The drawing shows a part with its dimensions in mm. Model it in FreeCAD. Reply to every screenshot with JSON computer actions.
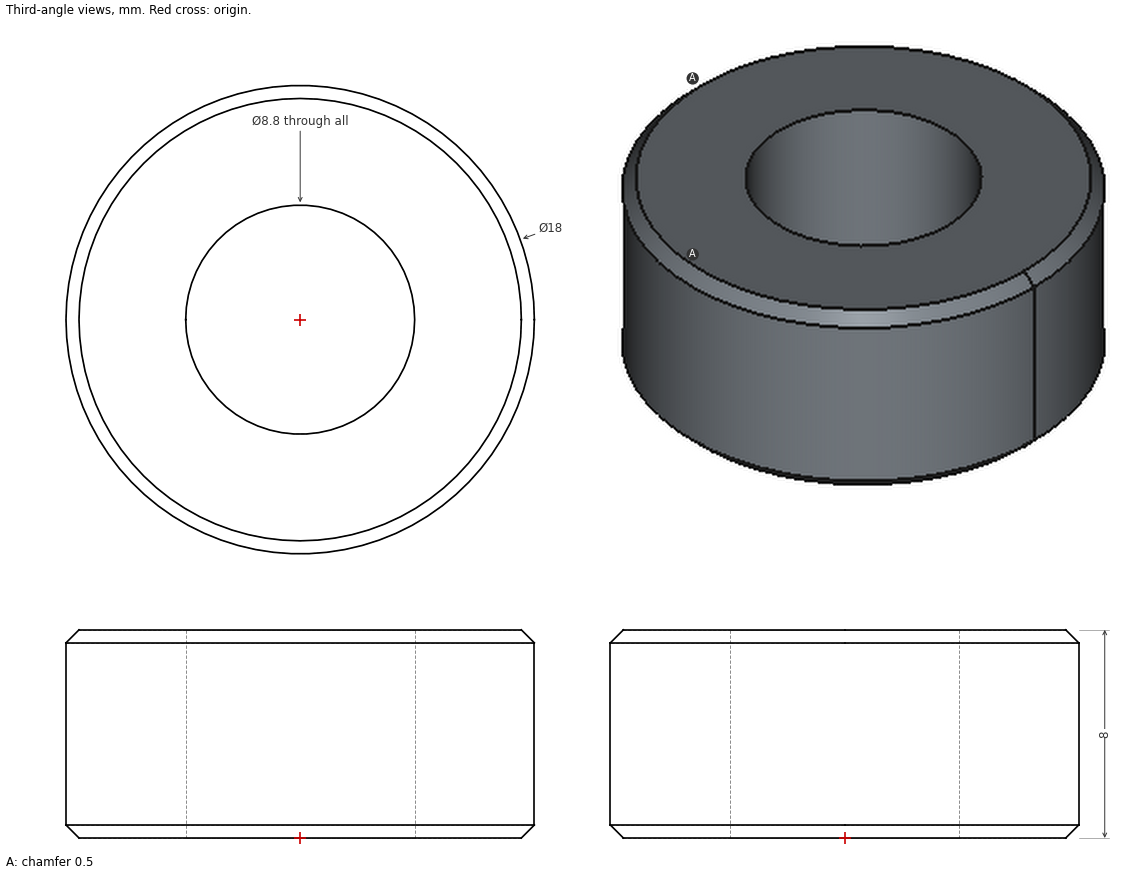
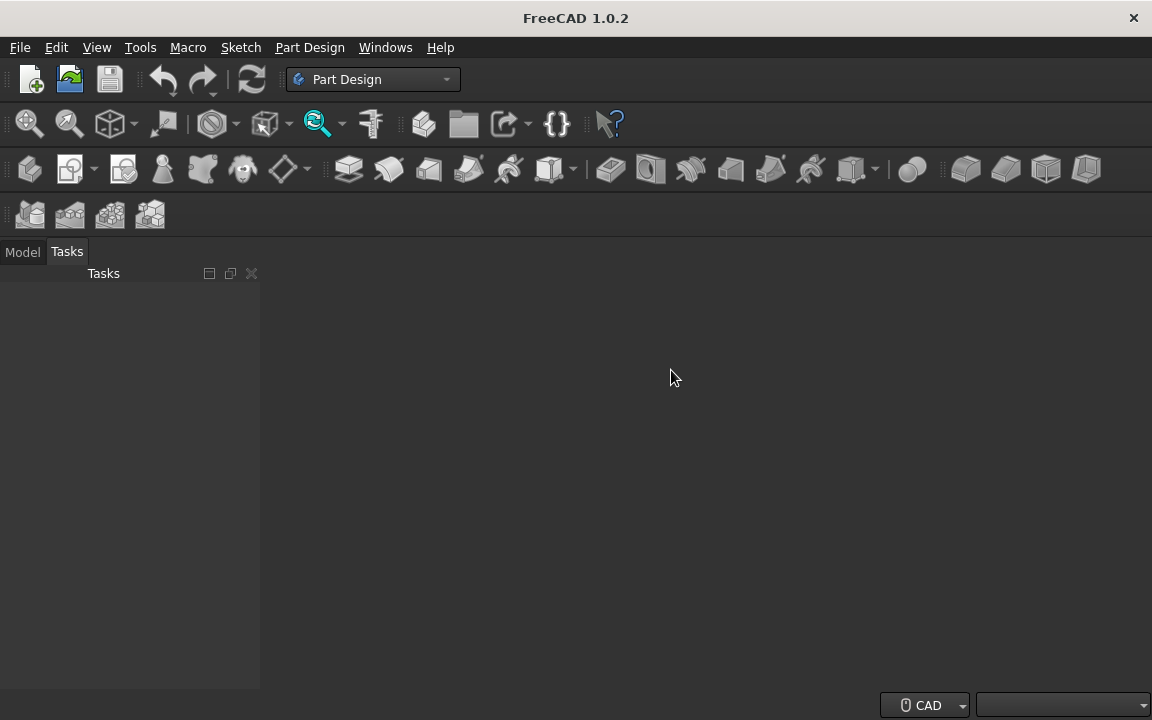
{"action": "left_click", "coordinate": [30, 80]}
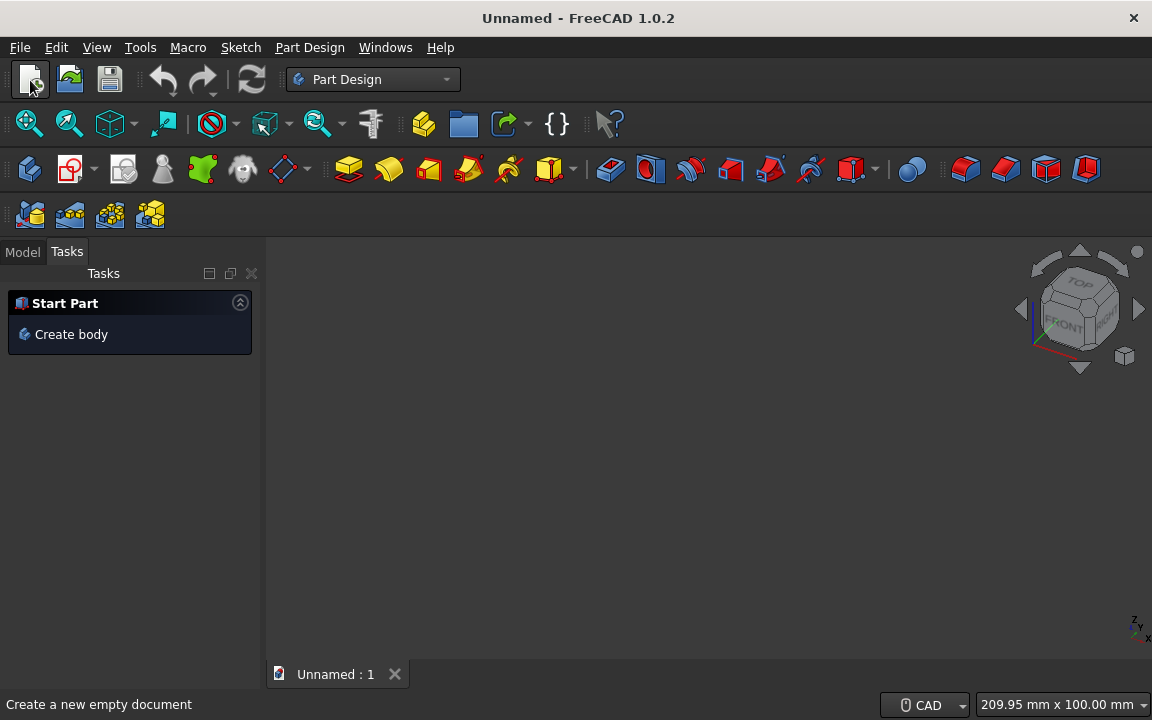
{"action": "left_click", "coordinate": [70, 170]}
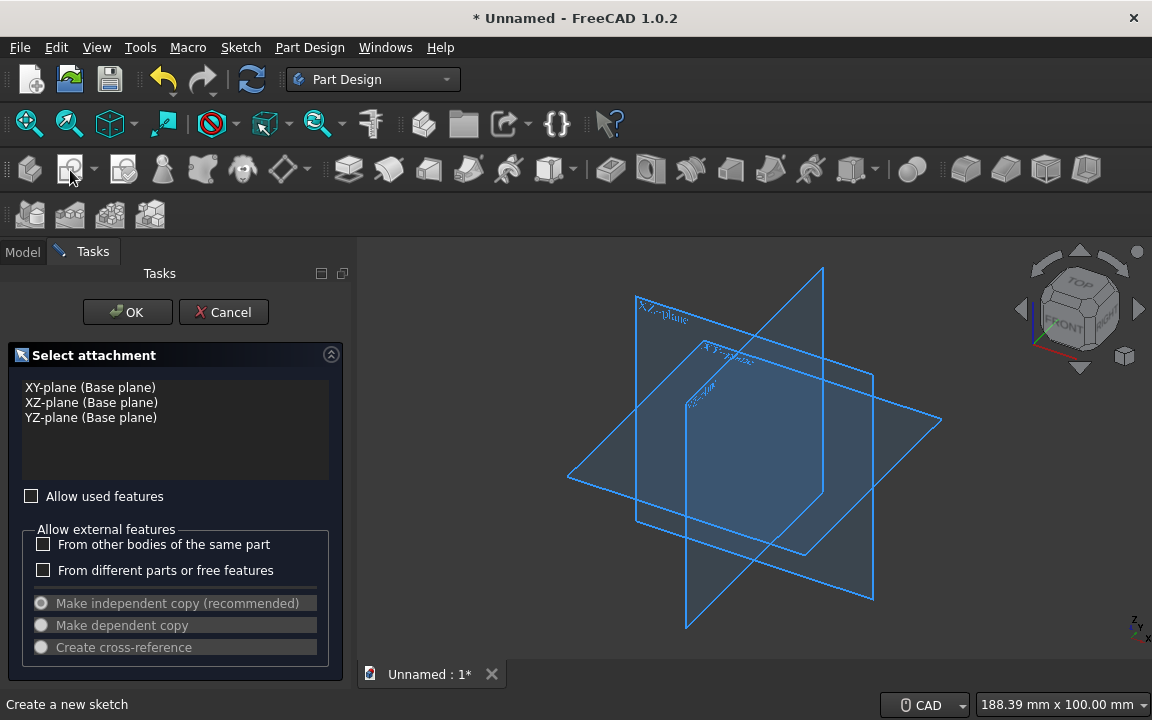
{"action": "left_click", "coordinate": [82, 388]}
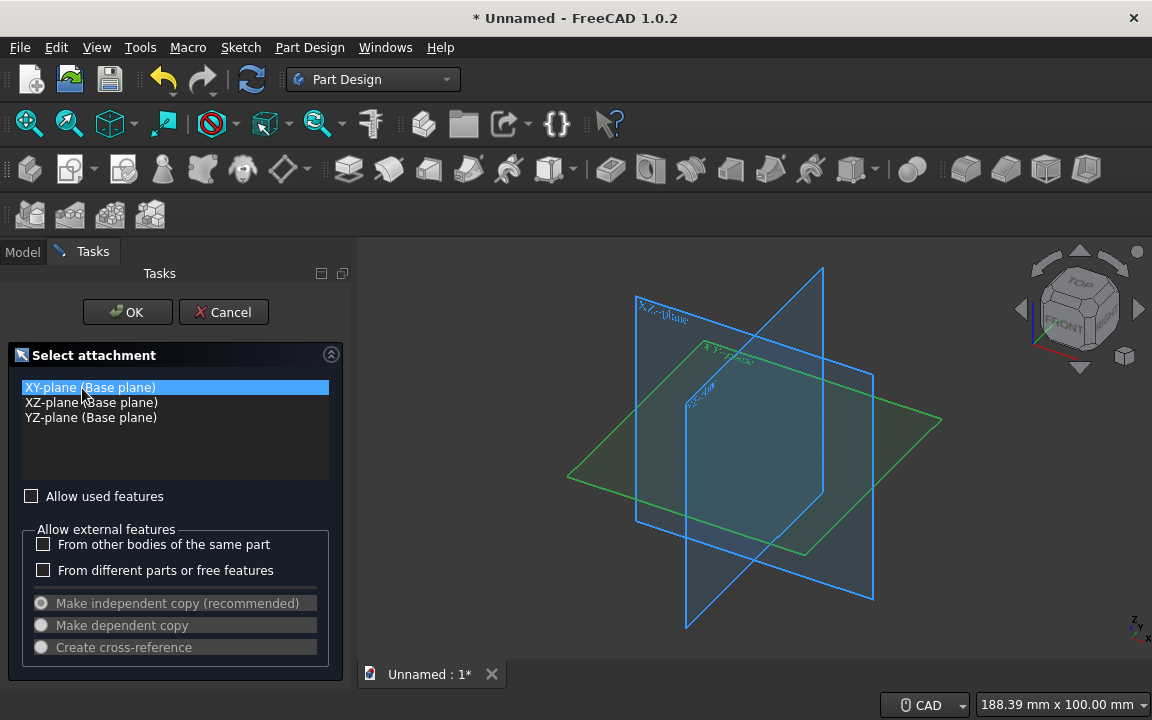
{"action": "left_click", "coordinate": [128, 312]}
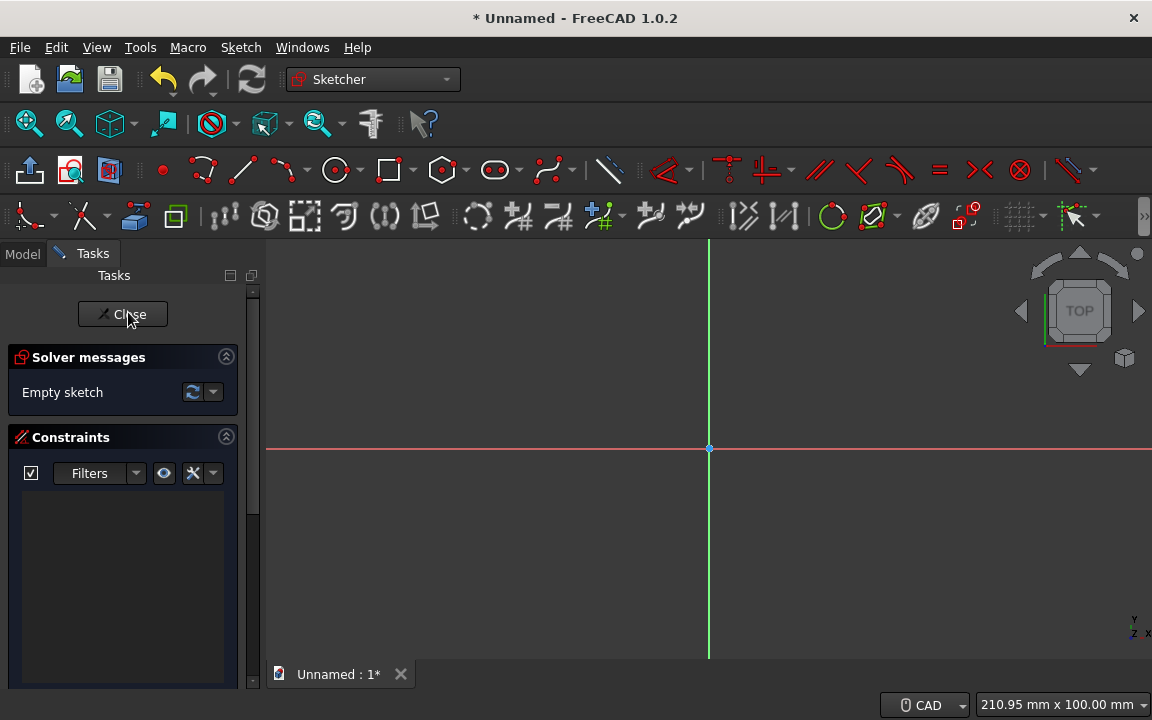
{"action": "scroll", "coordinate": [739, 449], "scroll_direction": "up", "scroll_amount": 6}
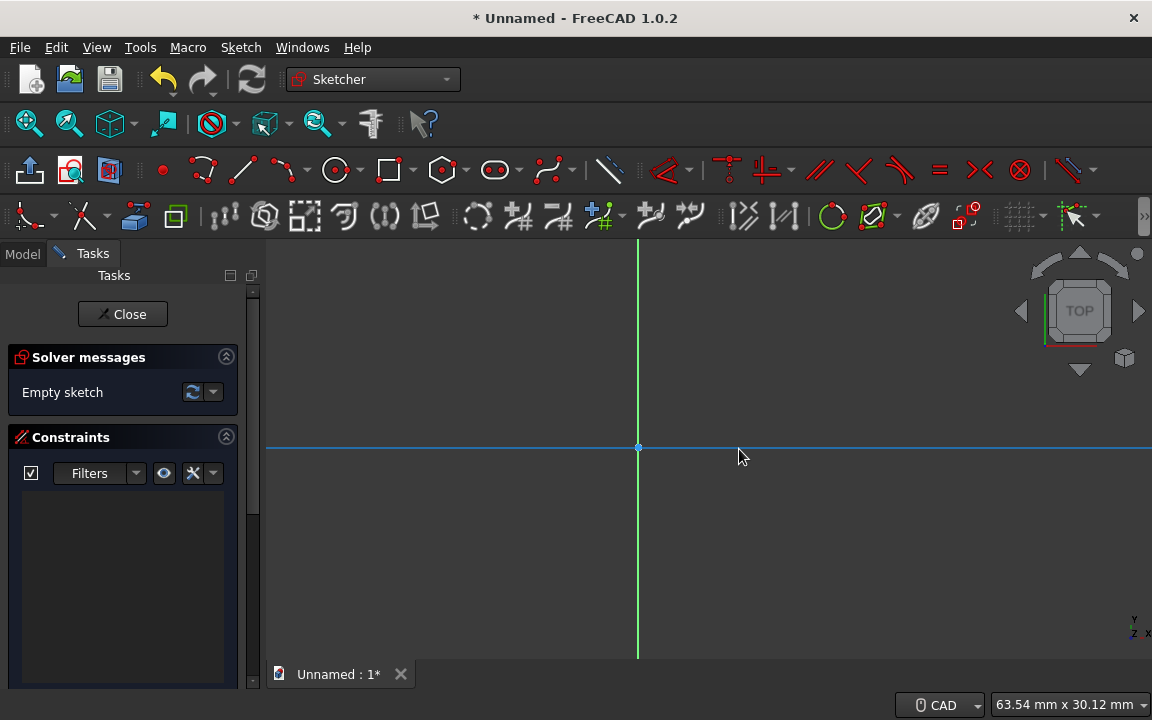
{"action": "left_click", "coordinate": [336, 170]}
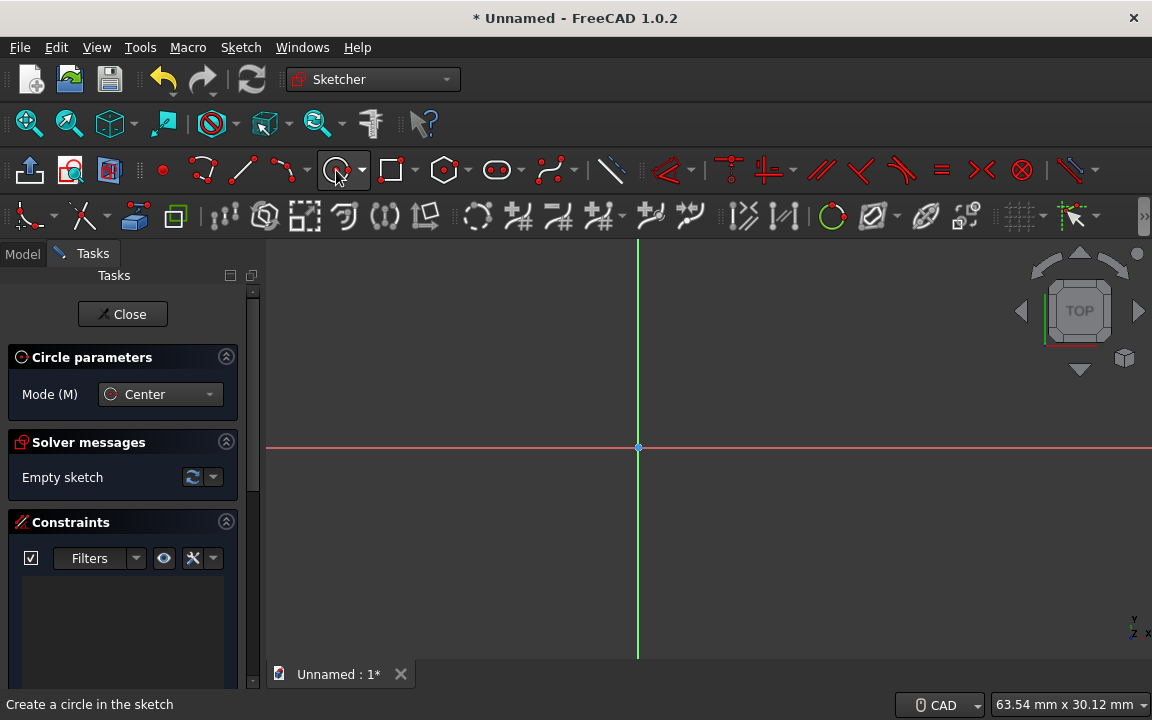
{"action": "left_click", "coordinate": [638, 448]}
{"action": "left_click", "coordinate": [727, 359]}
{"action": "key", "text": "Escape"}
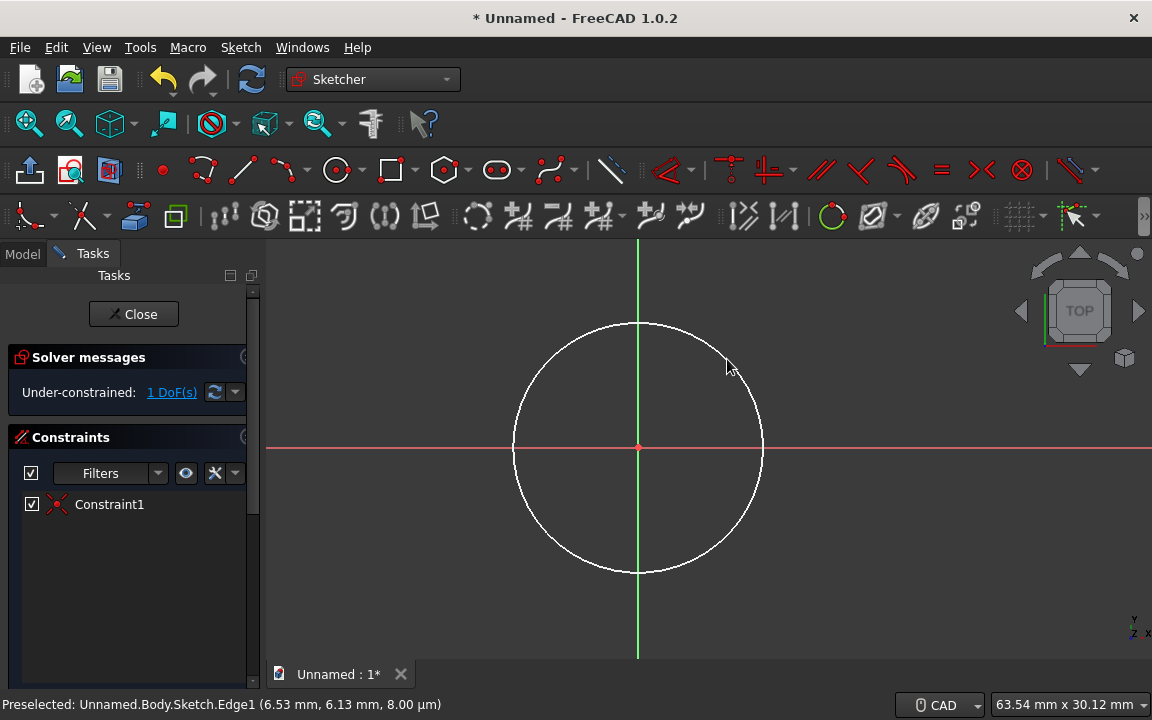
{"action": "key", "text": "d"}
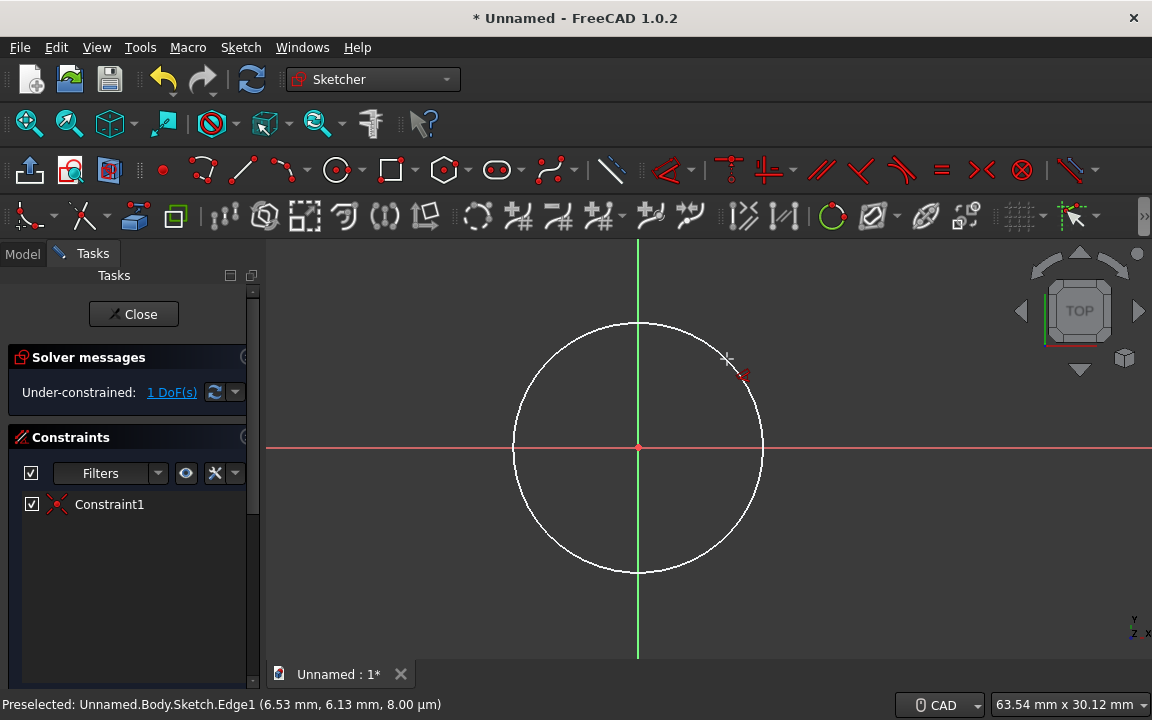
{"action": "left_click", "coordinate": [726, 359]}
{"action": "left_click", "coordinate": [748, 336]}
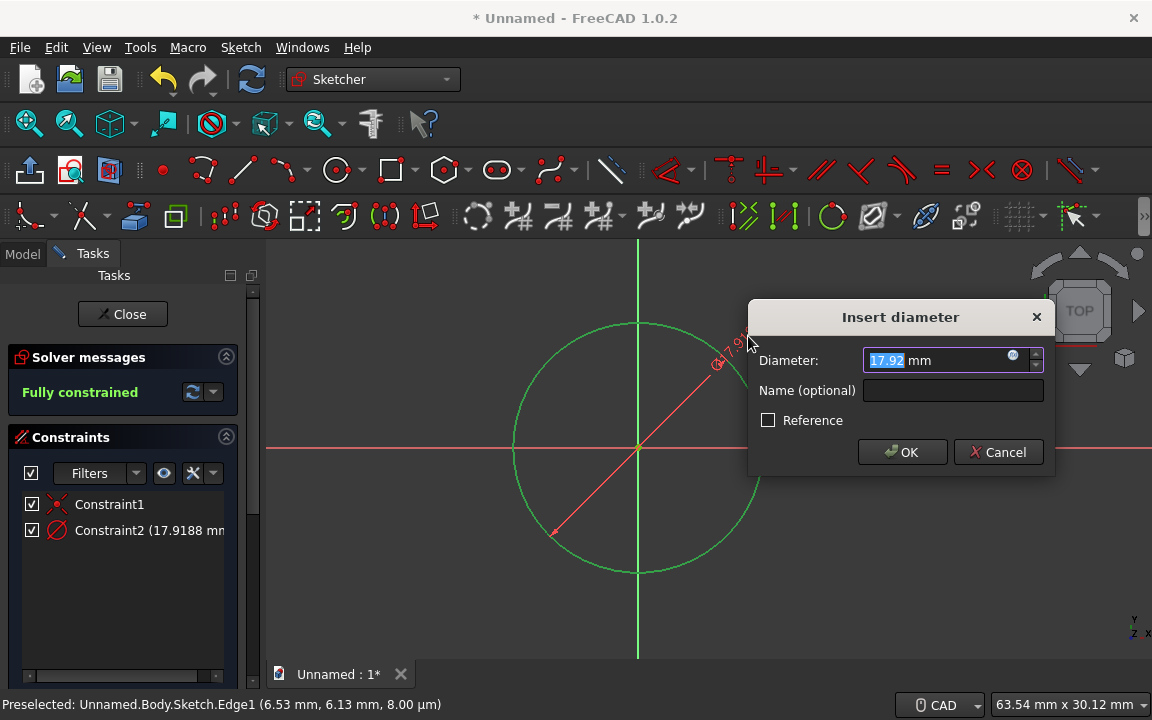
{"action": "type", "text": "18"}
{"action": "key", "text": "Return"}
{"action": "key", "text": "Escape"}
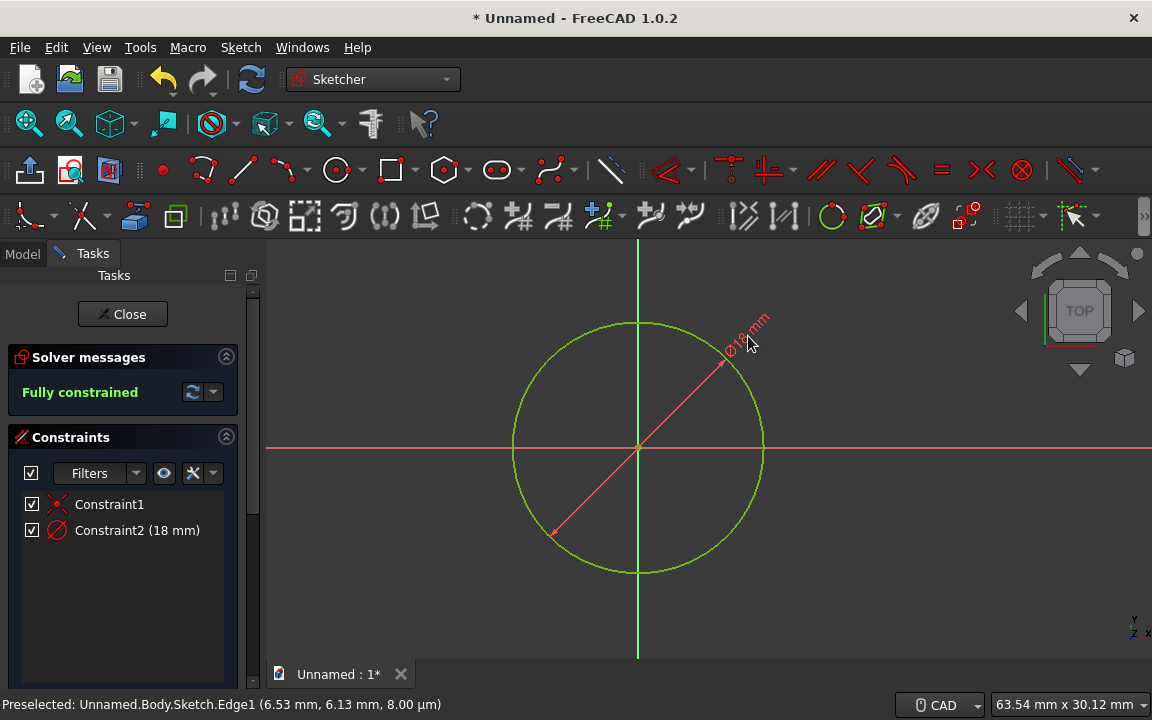
{"action": "left_click", "coordinate": [123, 314]}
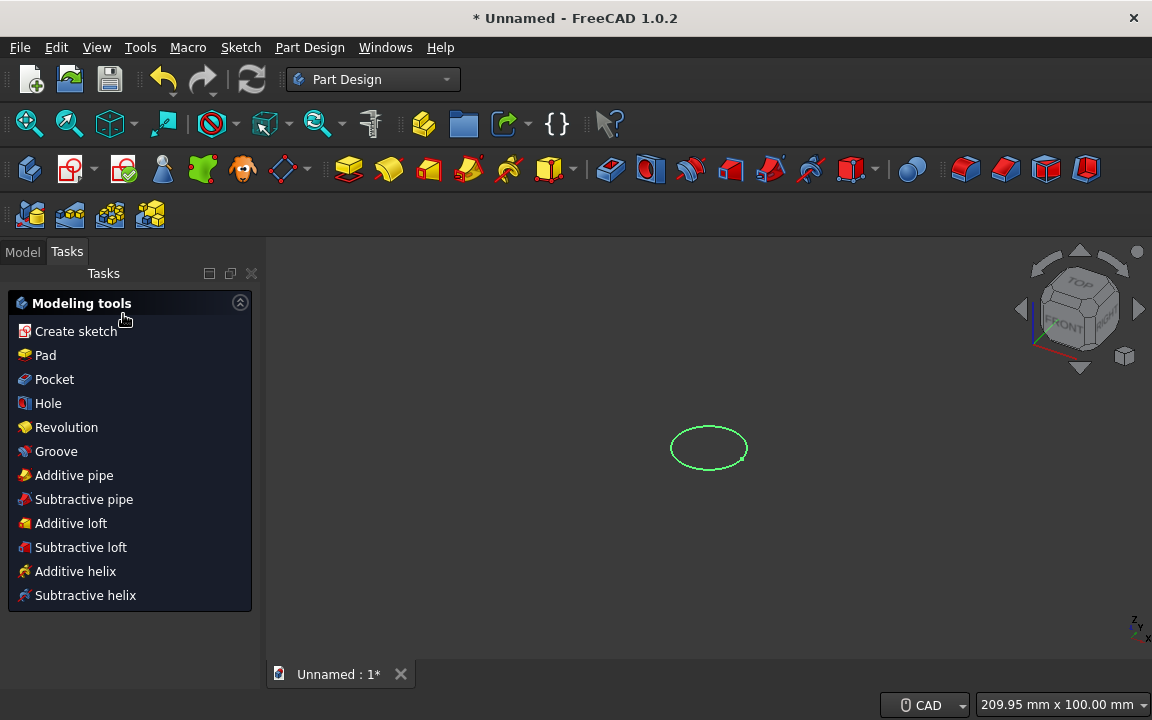
{"action": "left_click", "coordinate": [350, 170]}